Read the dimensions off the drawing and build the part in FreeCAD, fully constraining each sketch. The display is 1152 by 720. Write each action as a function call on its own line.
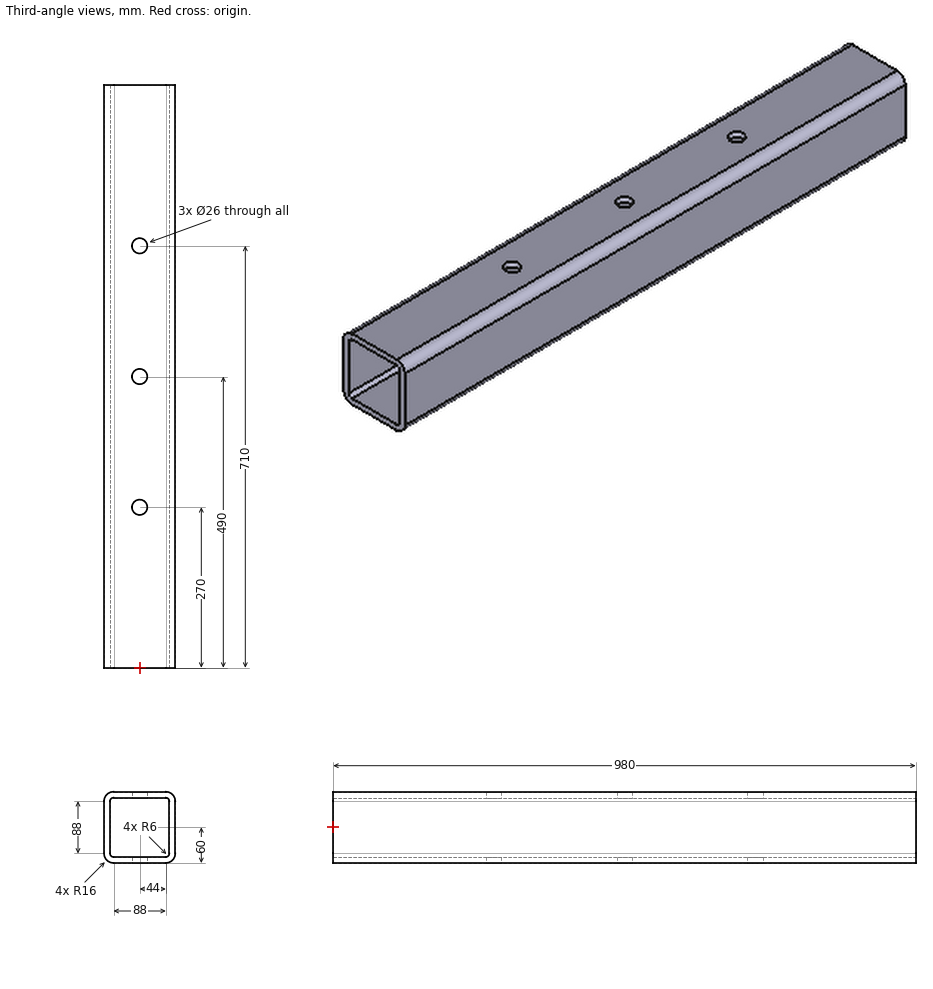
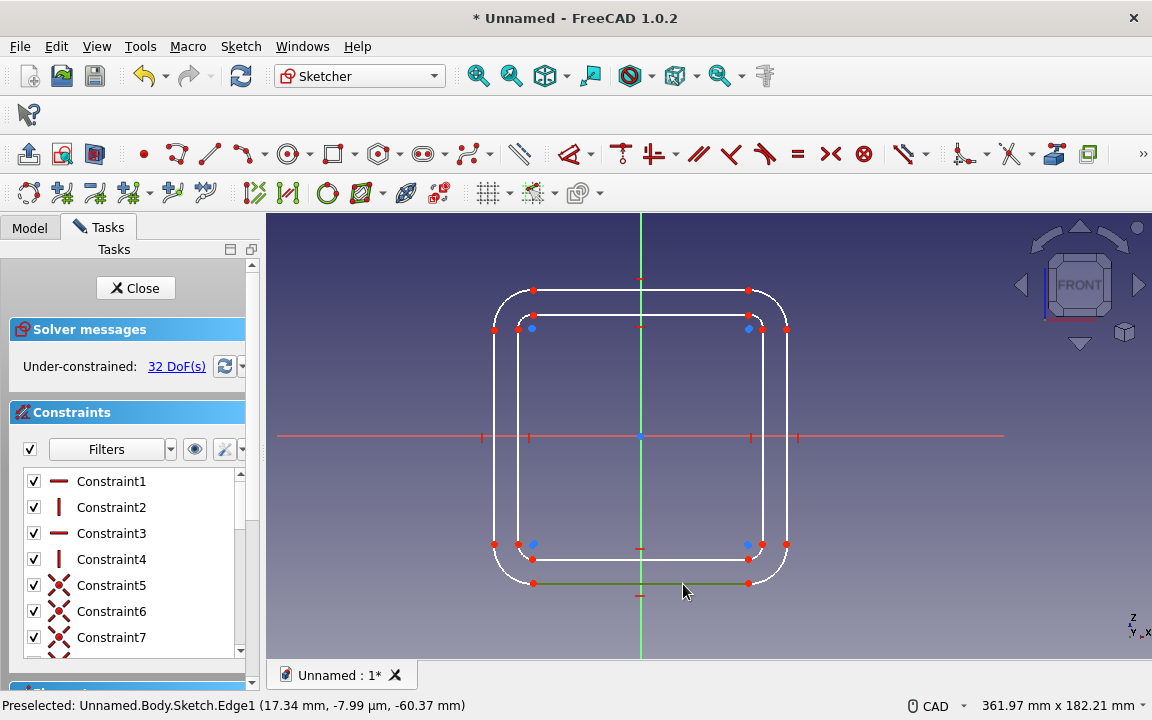
click(498, 563)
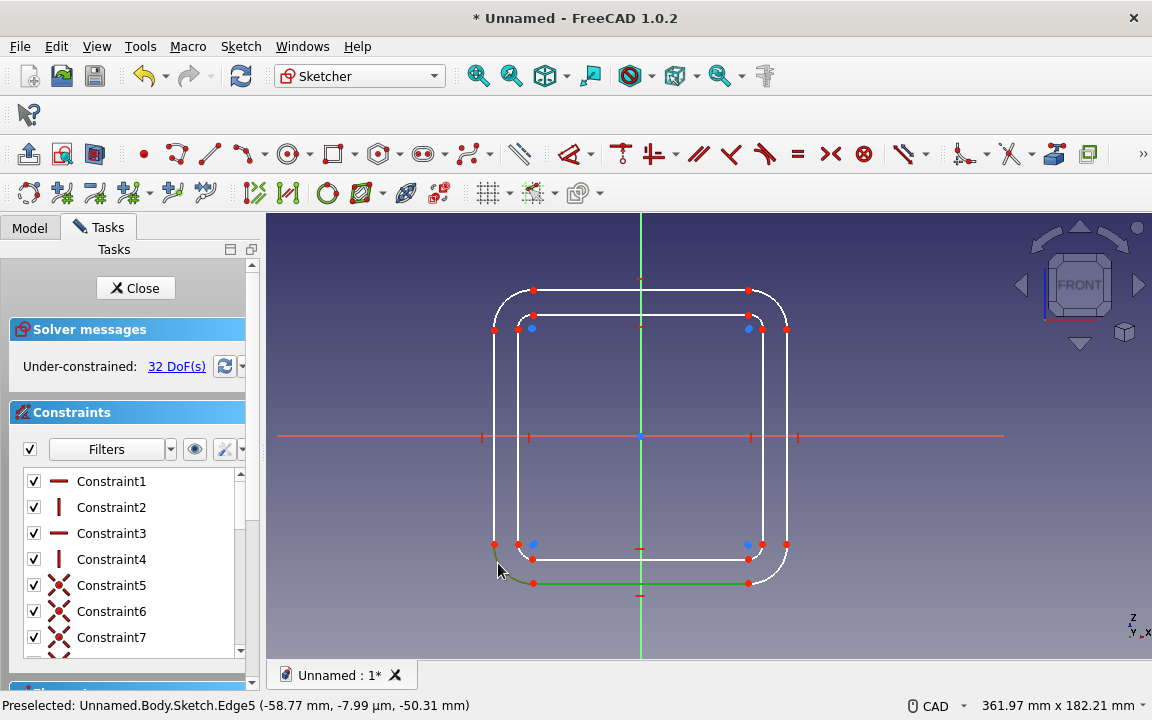
click(765, 154)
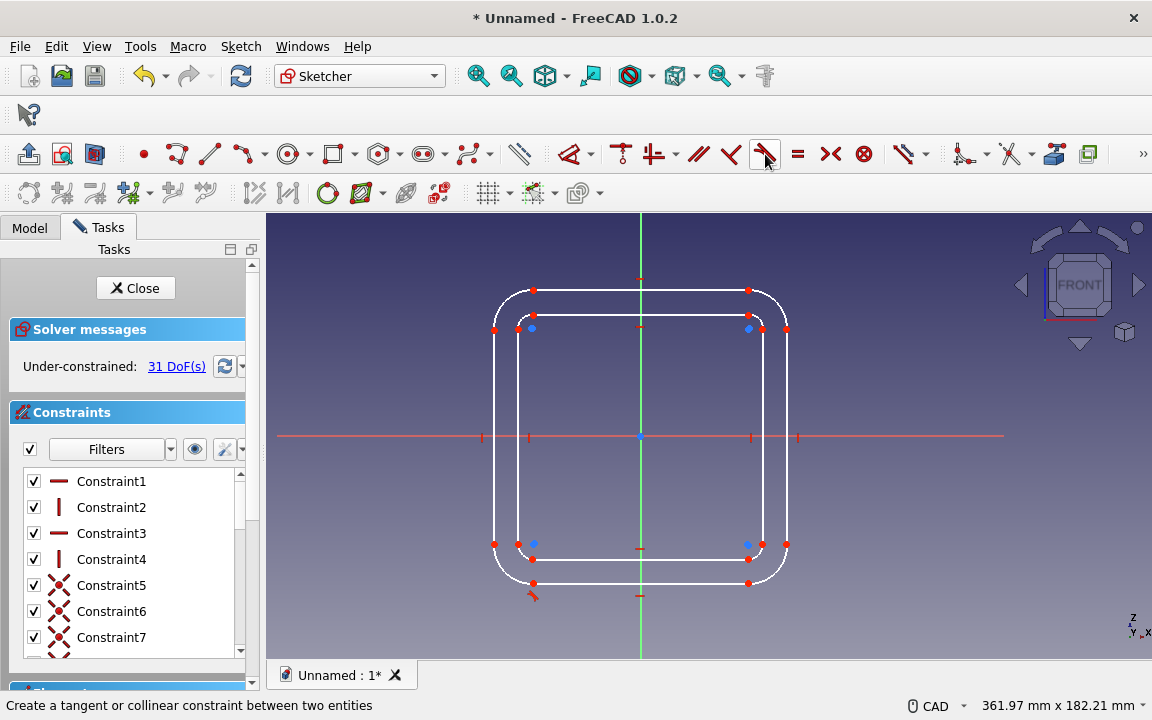
click(683, 584)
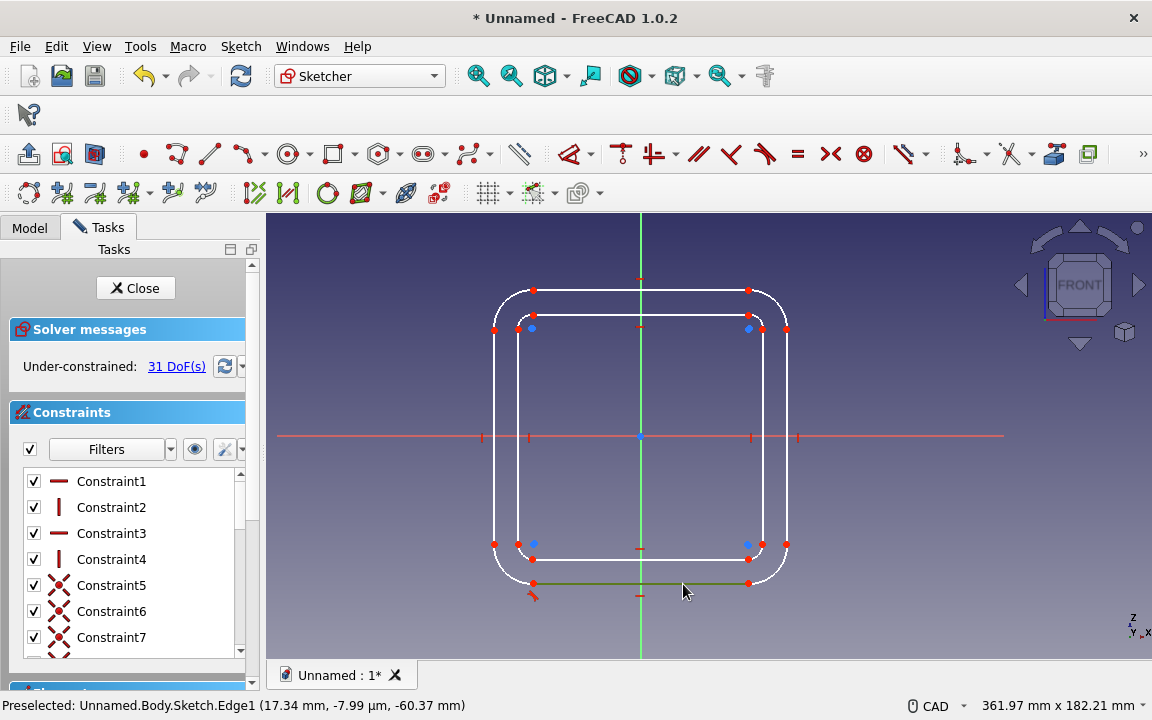
click(766, 580)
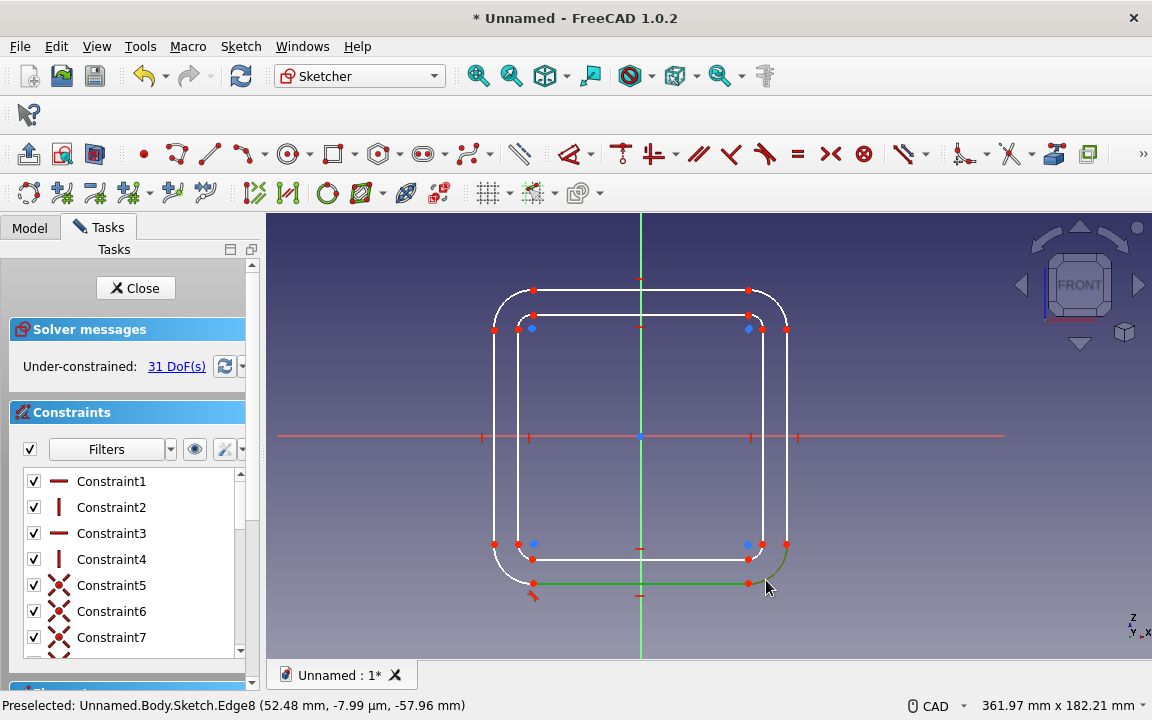
click(765, 154)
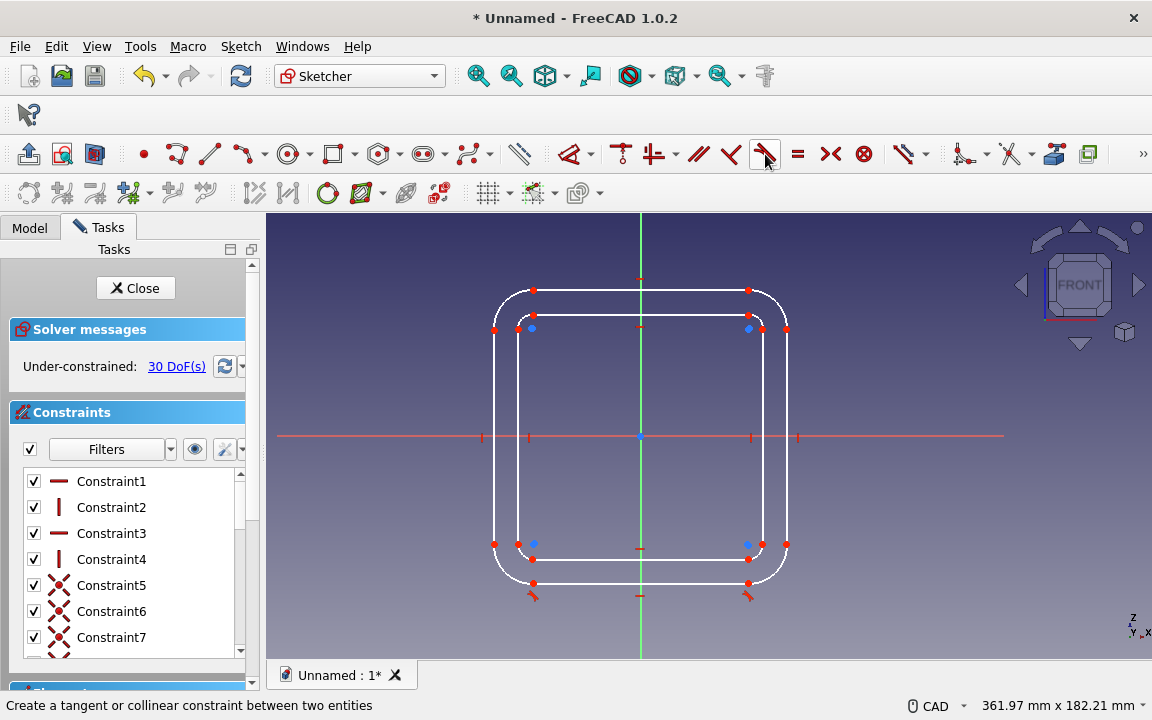
click(494, 481)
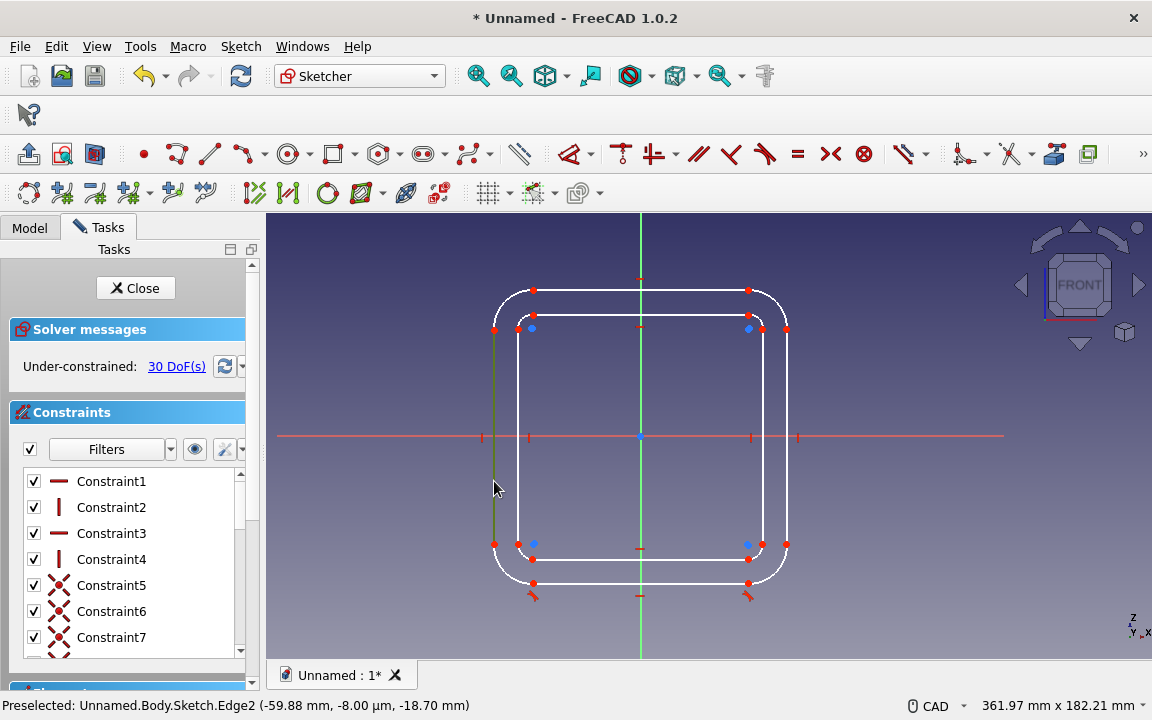
click(498, 563)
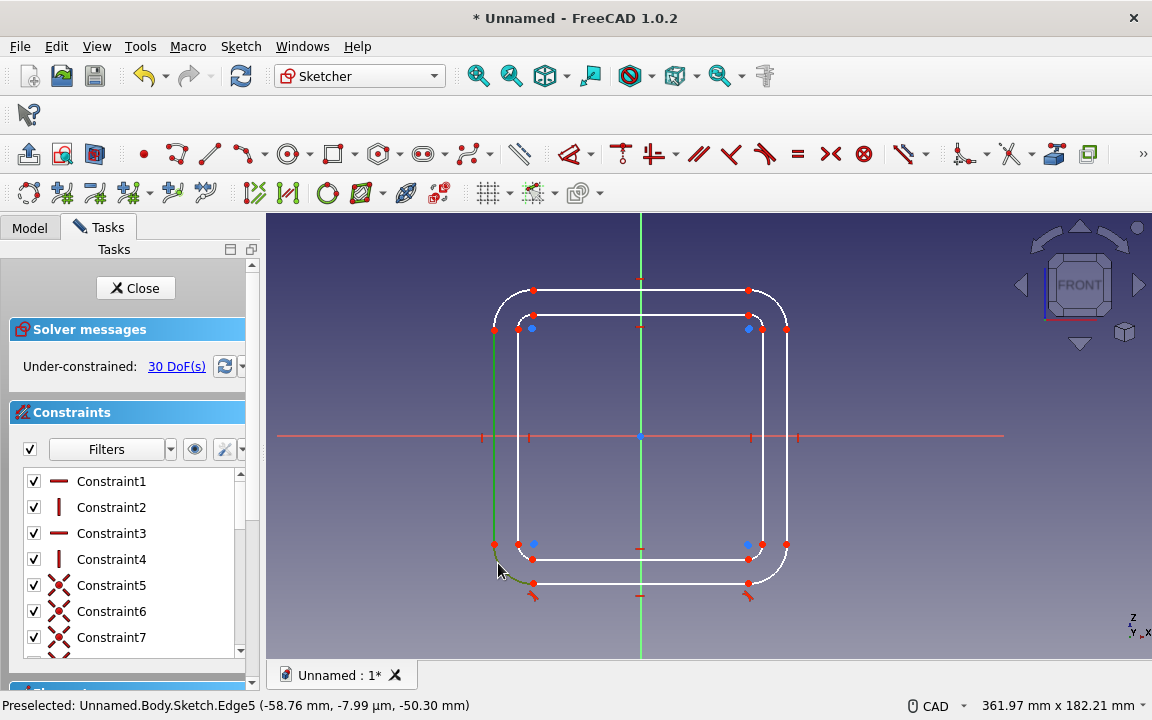
click(765, 154)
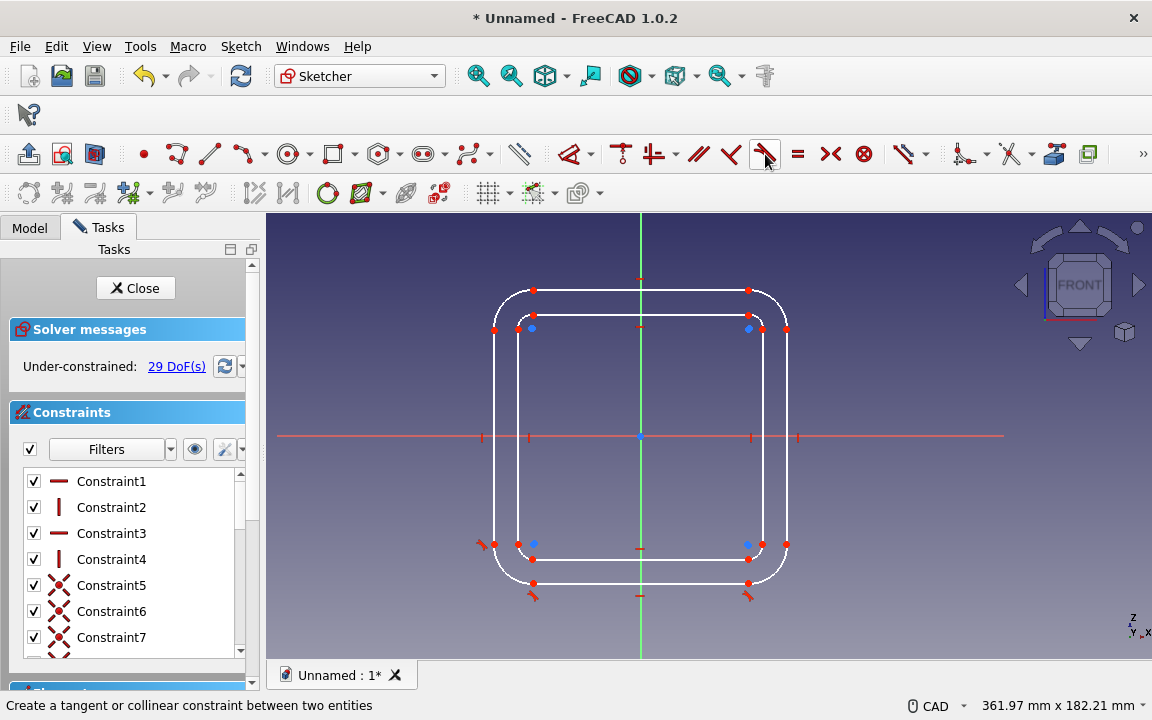
click(494, 481)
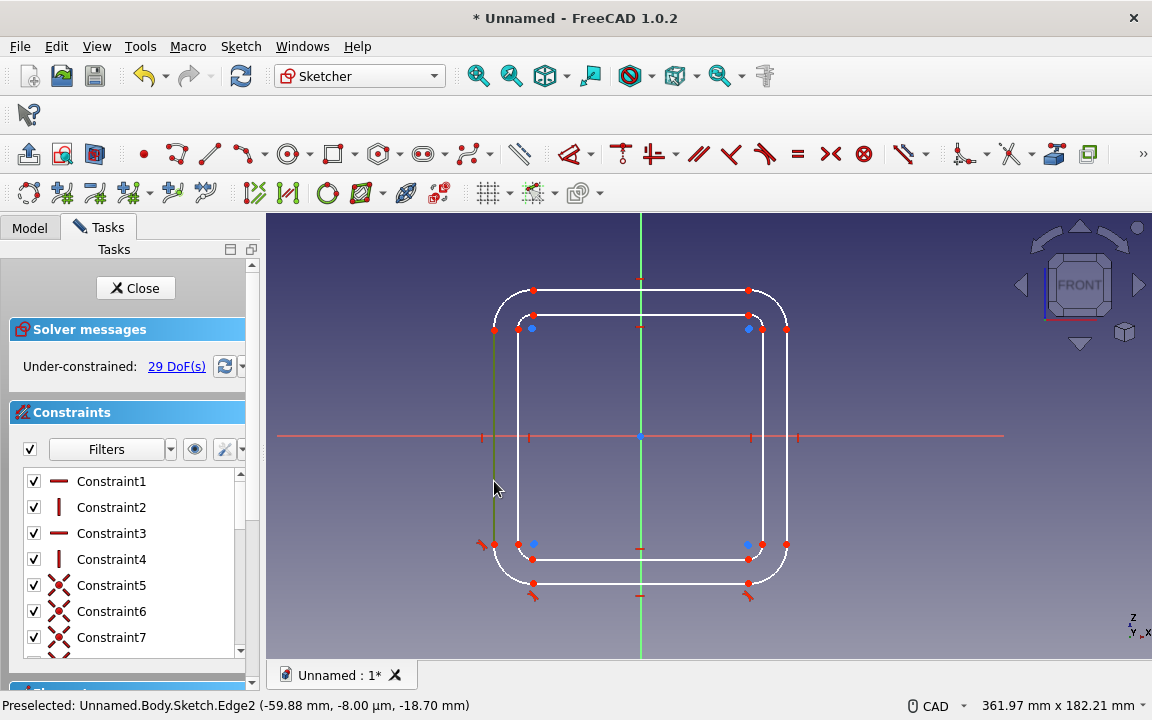
click(515, 294)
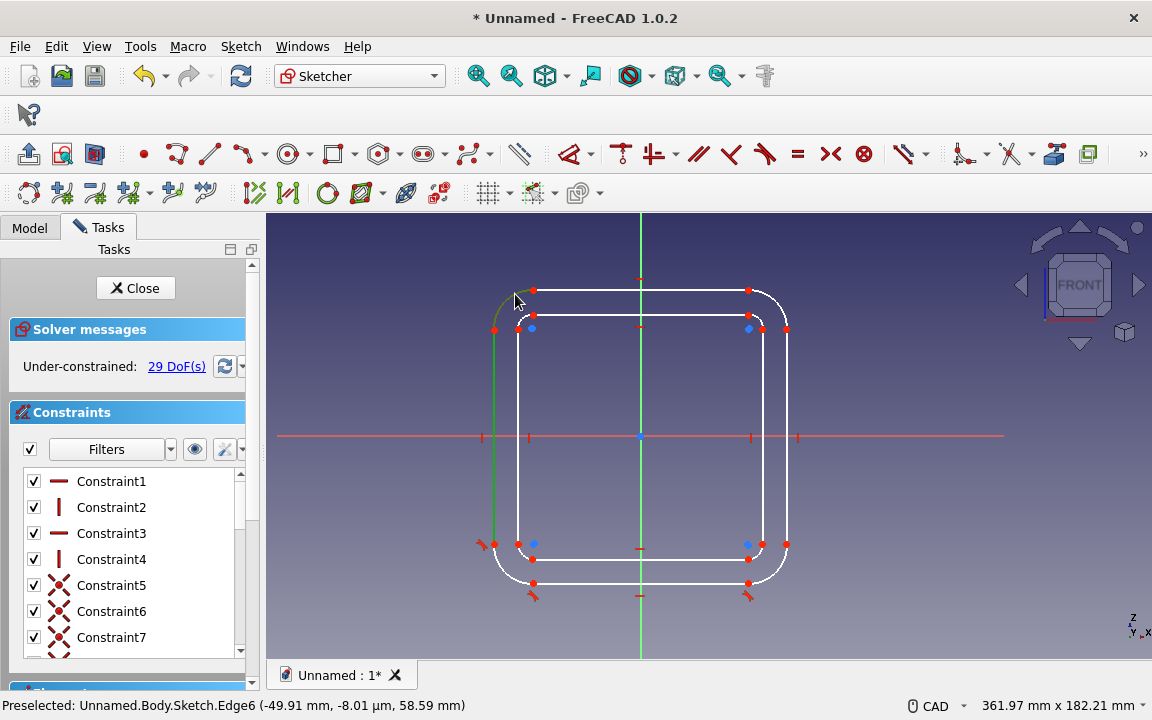
click(765, 154)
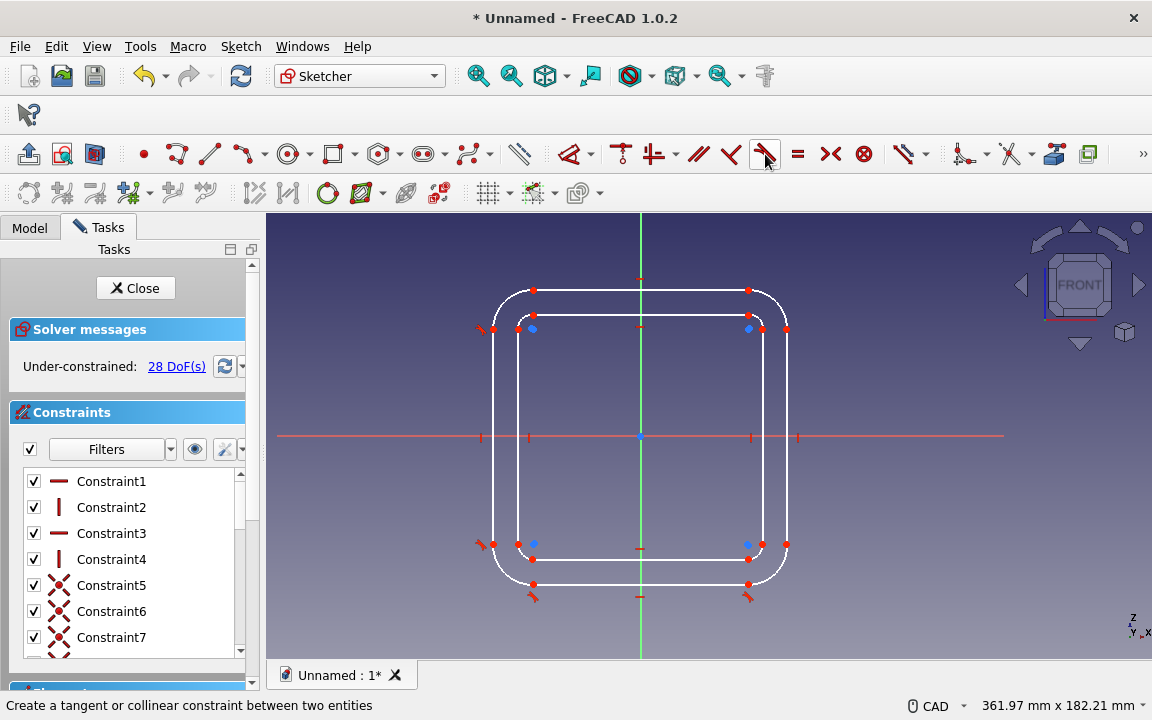
click(598, 290)